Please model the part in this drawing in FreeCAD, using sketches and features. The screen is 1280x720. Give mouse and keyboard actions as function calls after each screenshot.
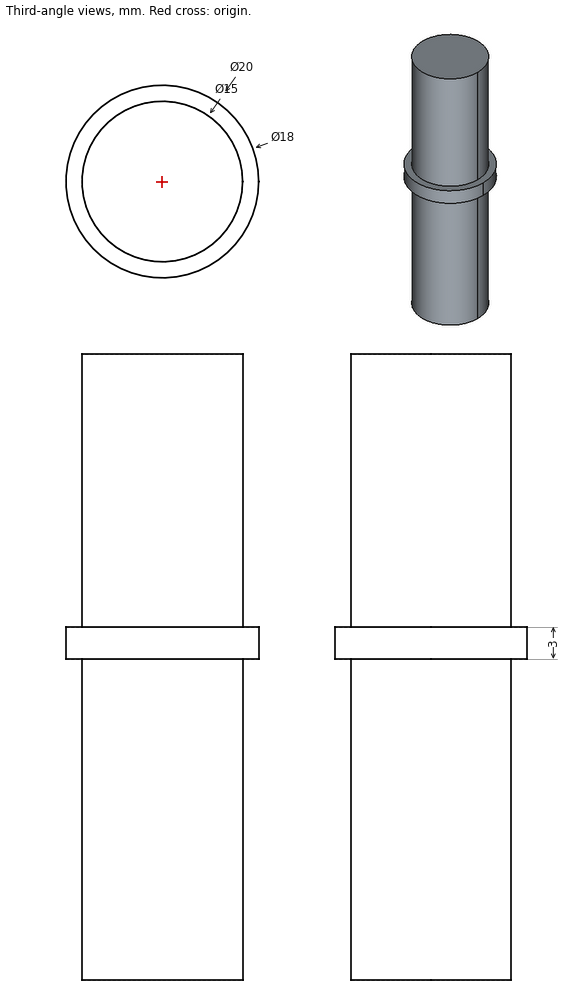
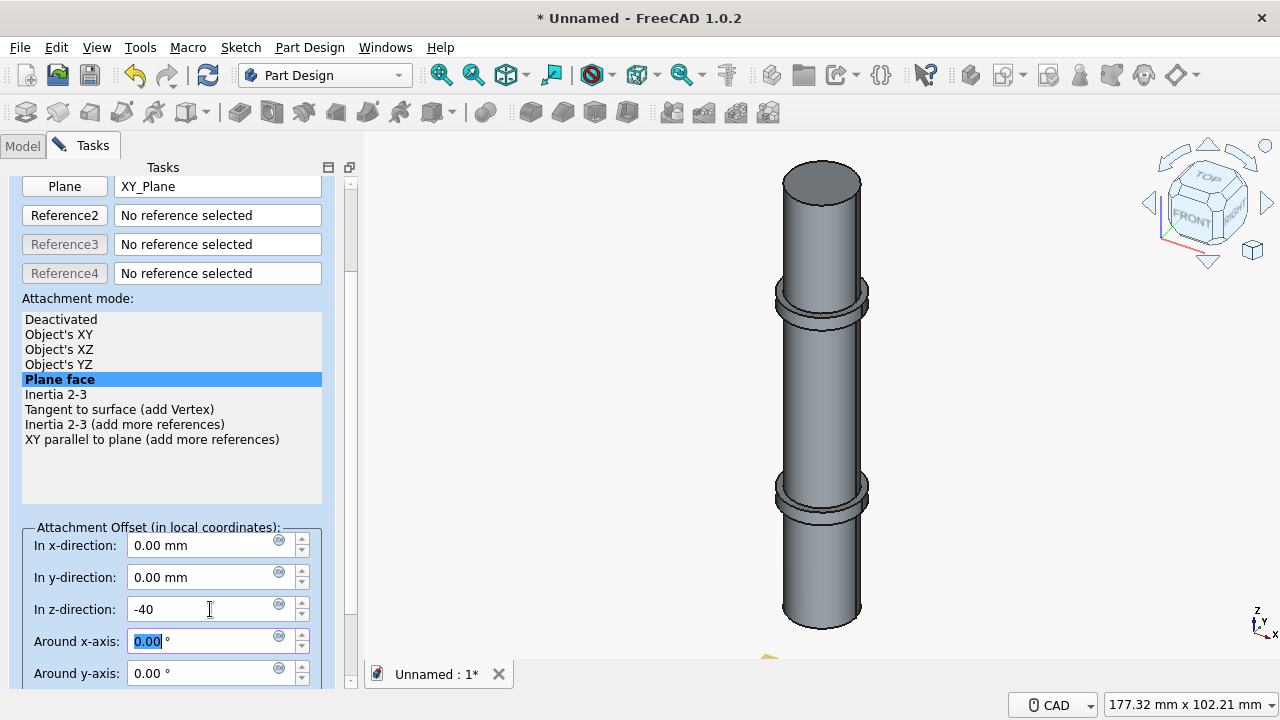
scroll(351, 432, up, 3)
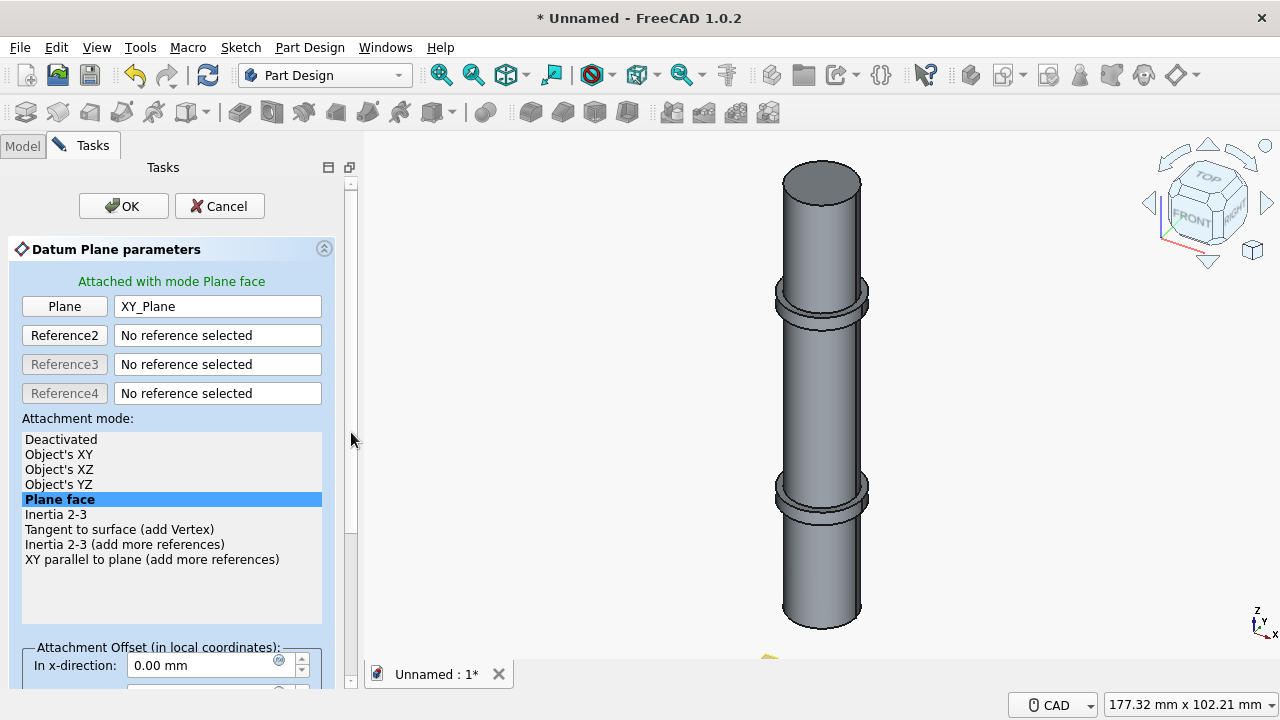
click(124, 206)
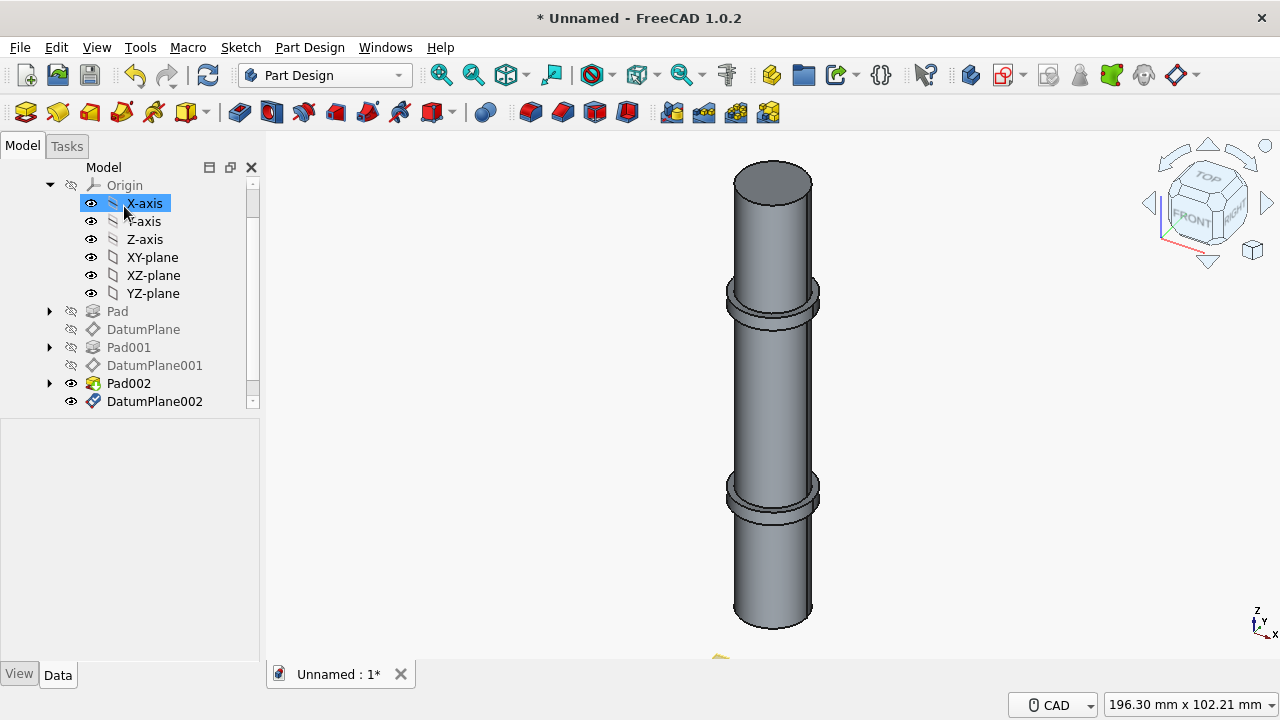
click(116, 401)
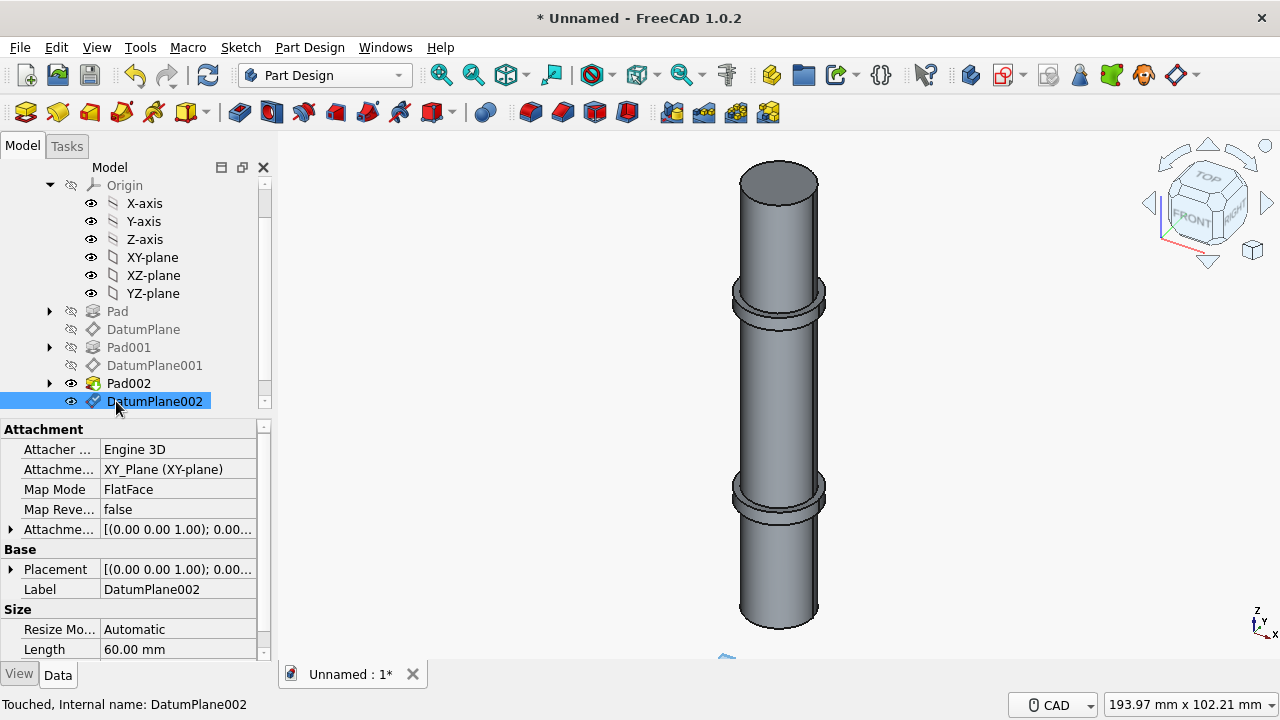
click(1004, 76)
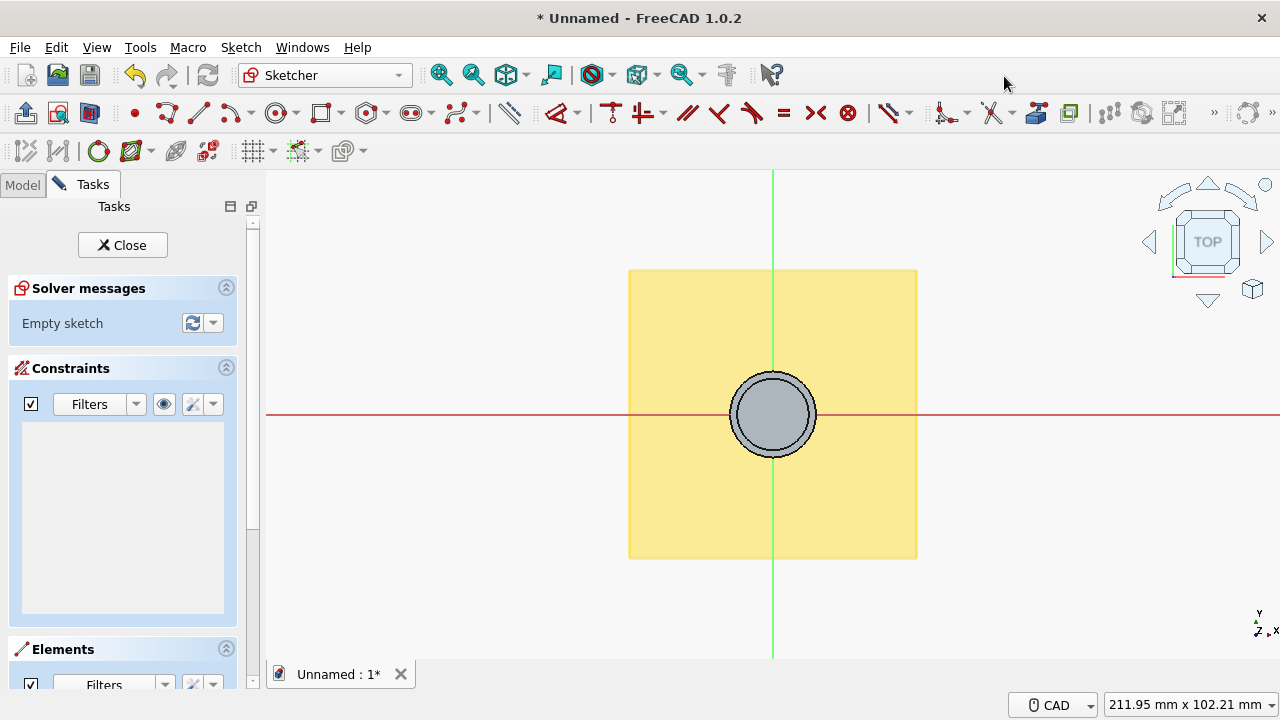
click(90, 114)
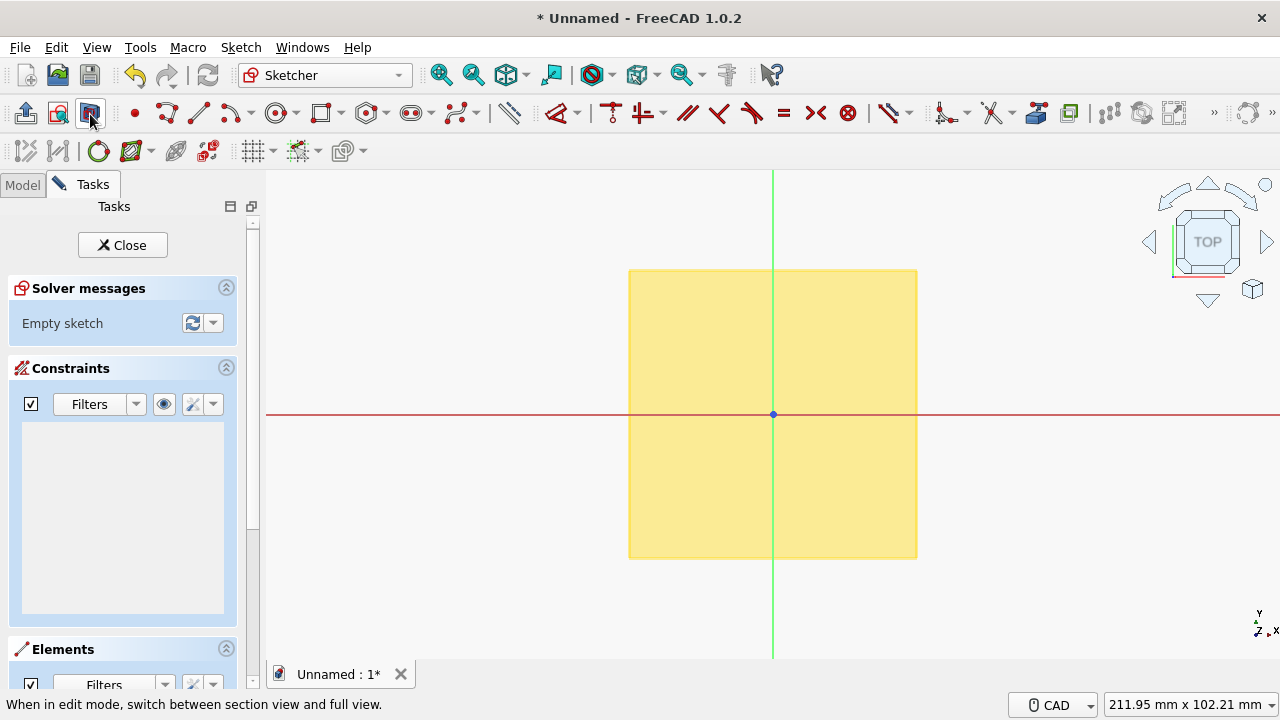
scroll(795, 415, up, 7)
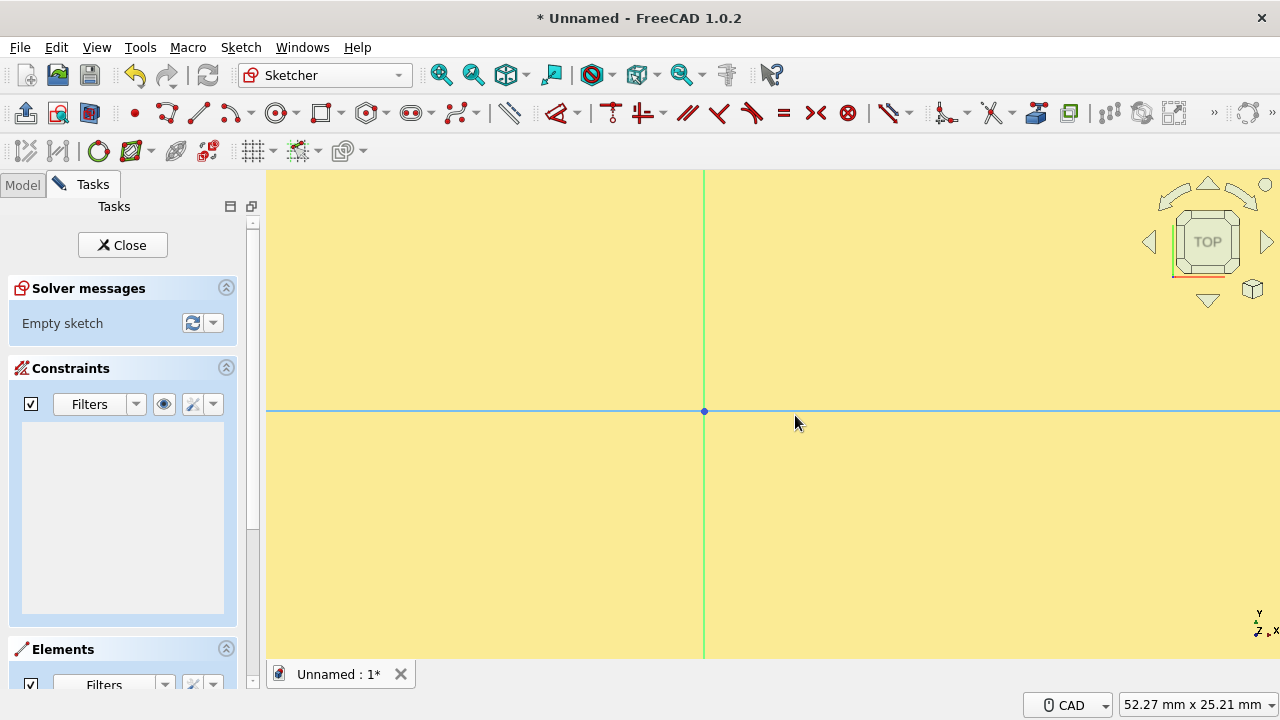
click(276, 114)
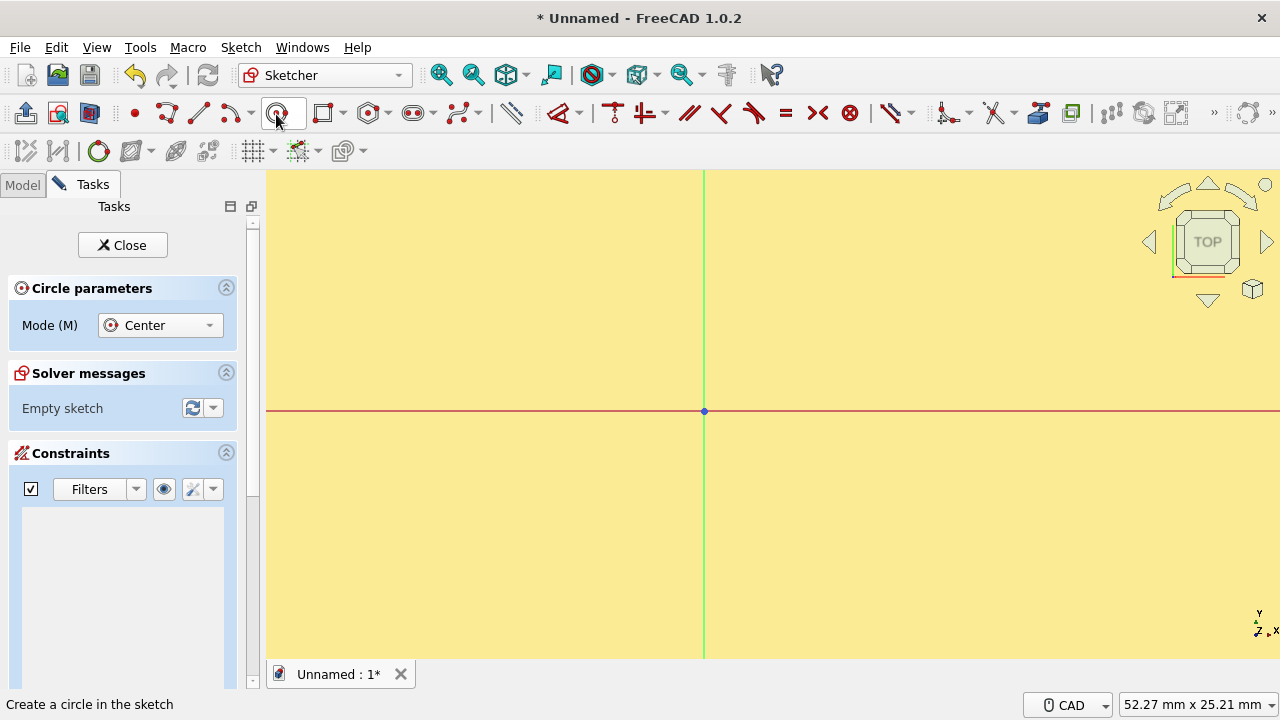
click(704, 411)
click(807, 309)
key(Escape)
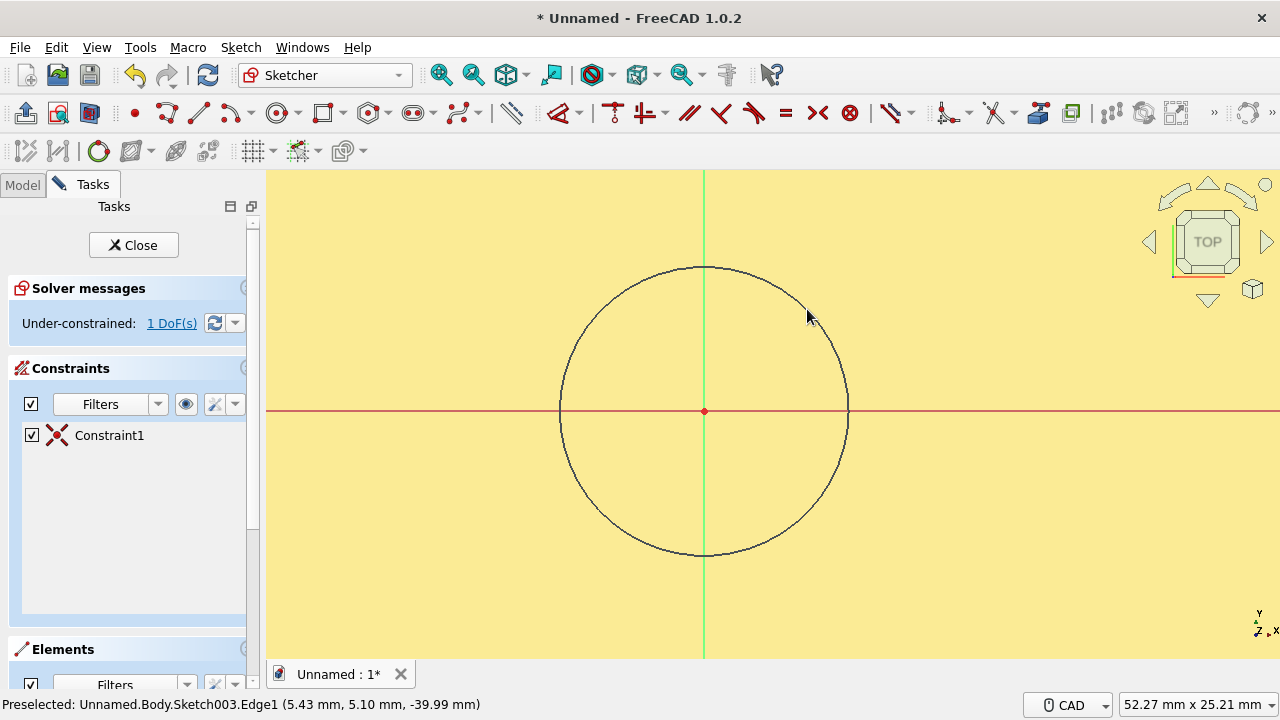
click(558, 114)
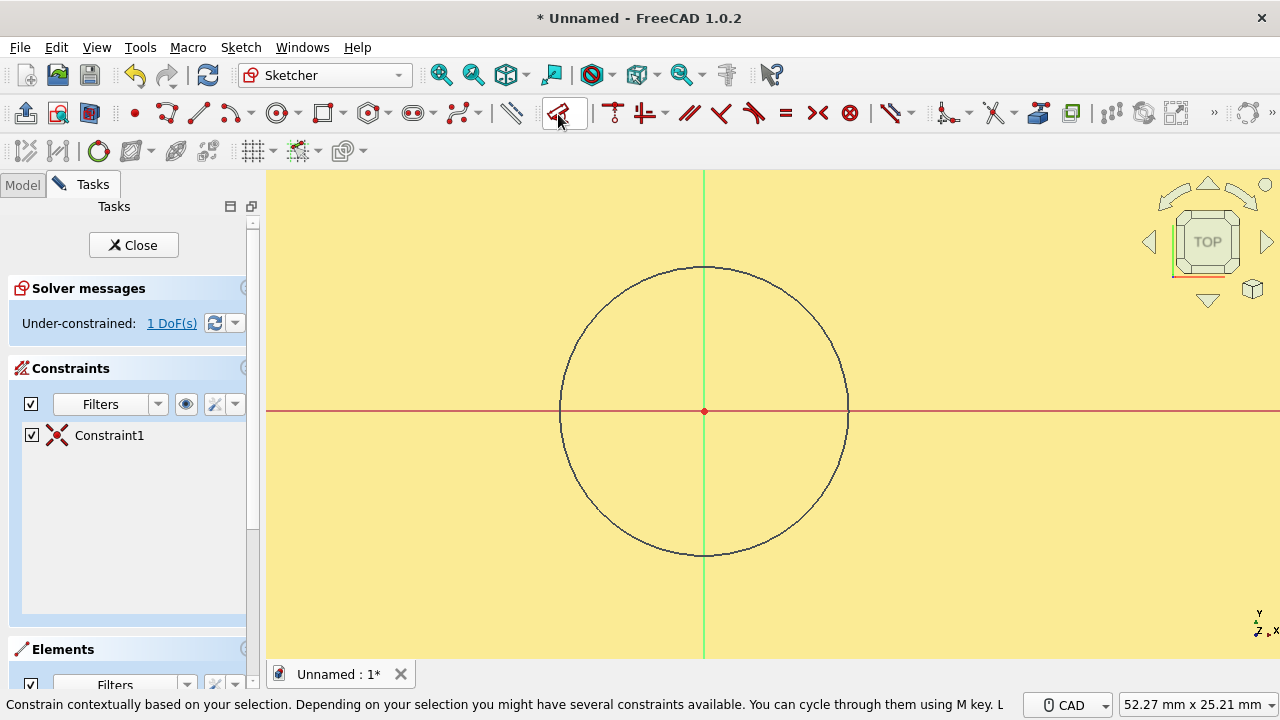
click(806, 309)
click(829, 286)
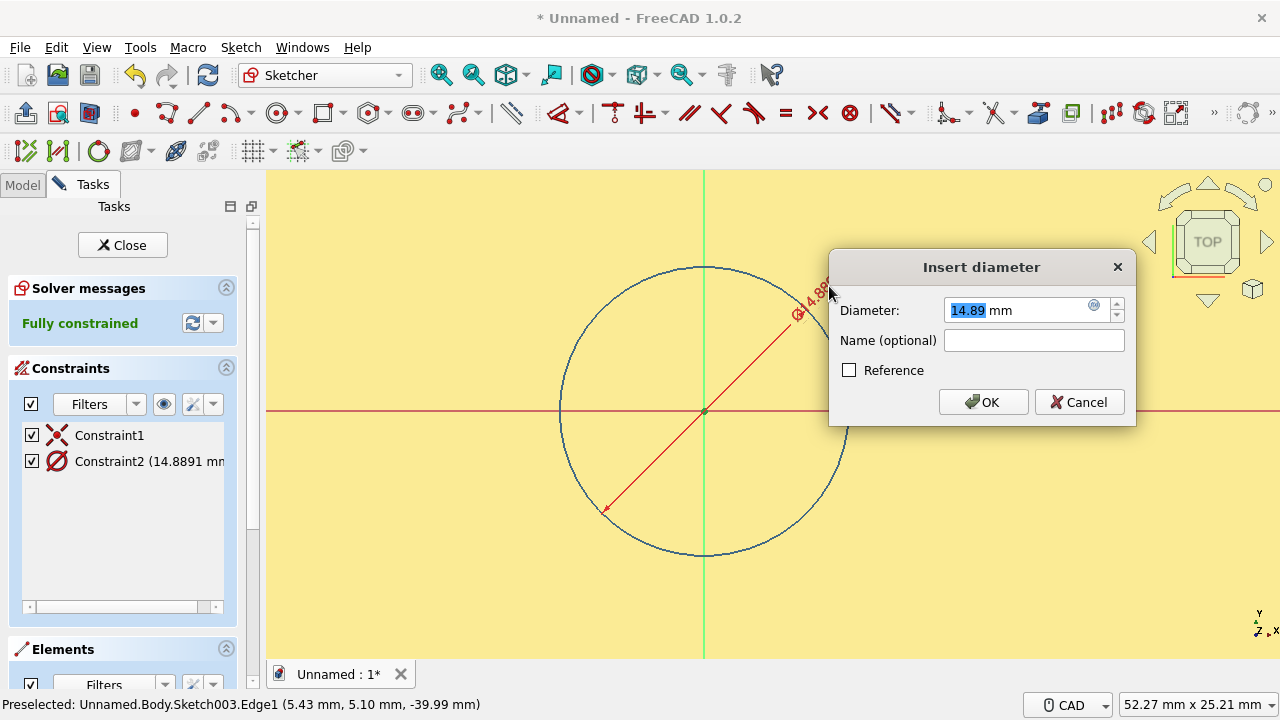
text(15)
key(Return)
key(Escape)